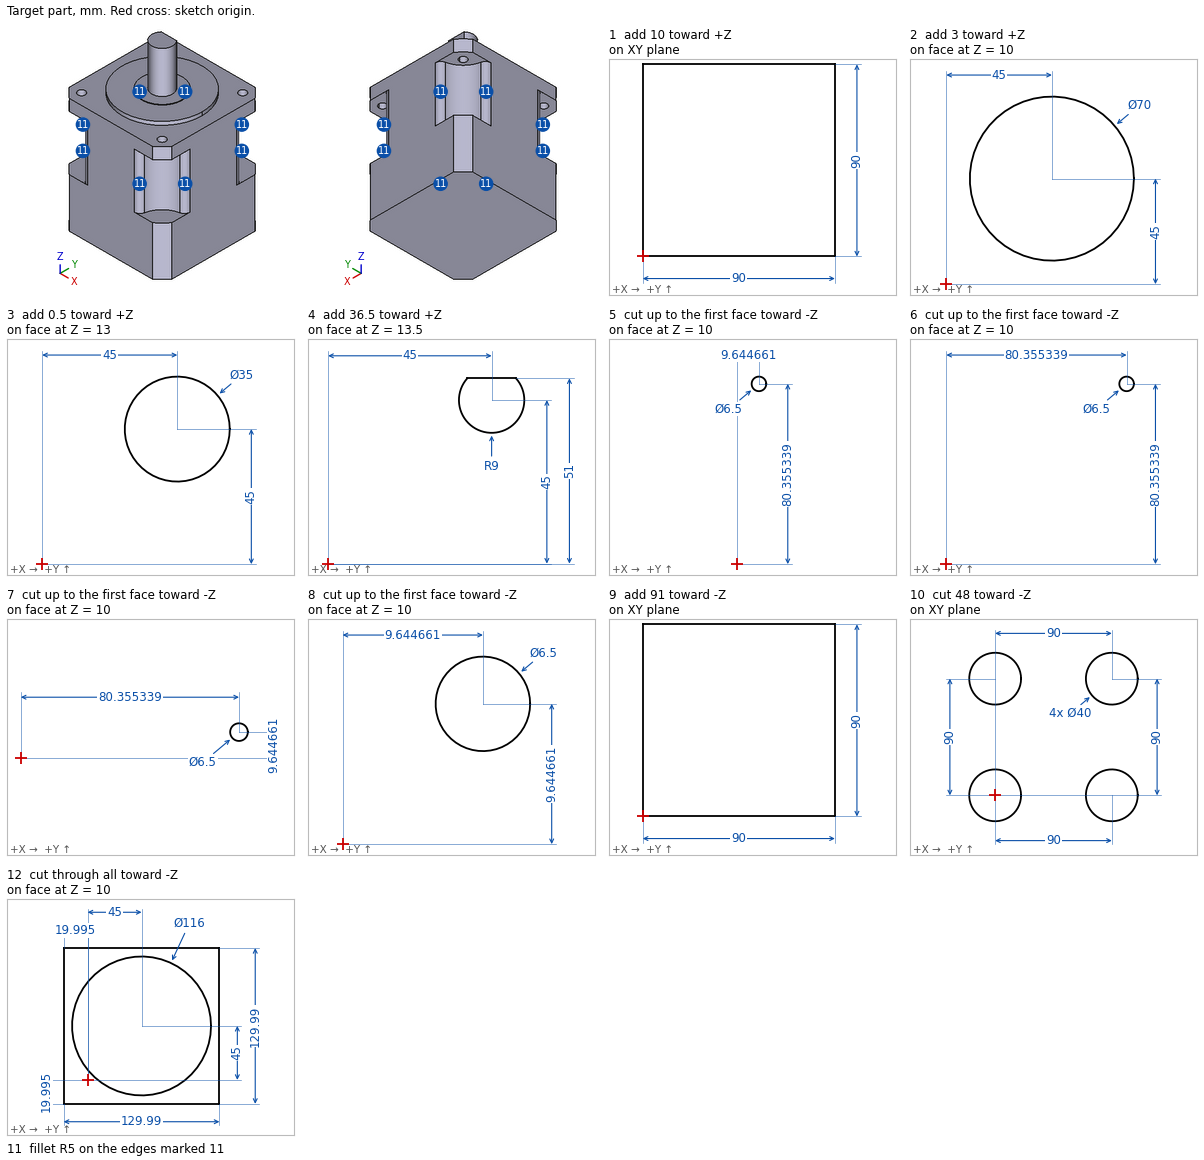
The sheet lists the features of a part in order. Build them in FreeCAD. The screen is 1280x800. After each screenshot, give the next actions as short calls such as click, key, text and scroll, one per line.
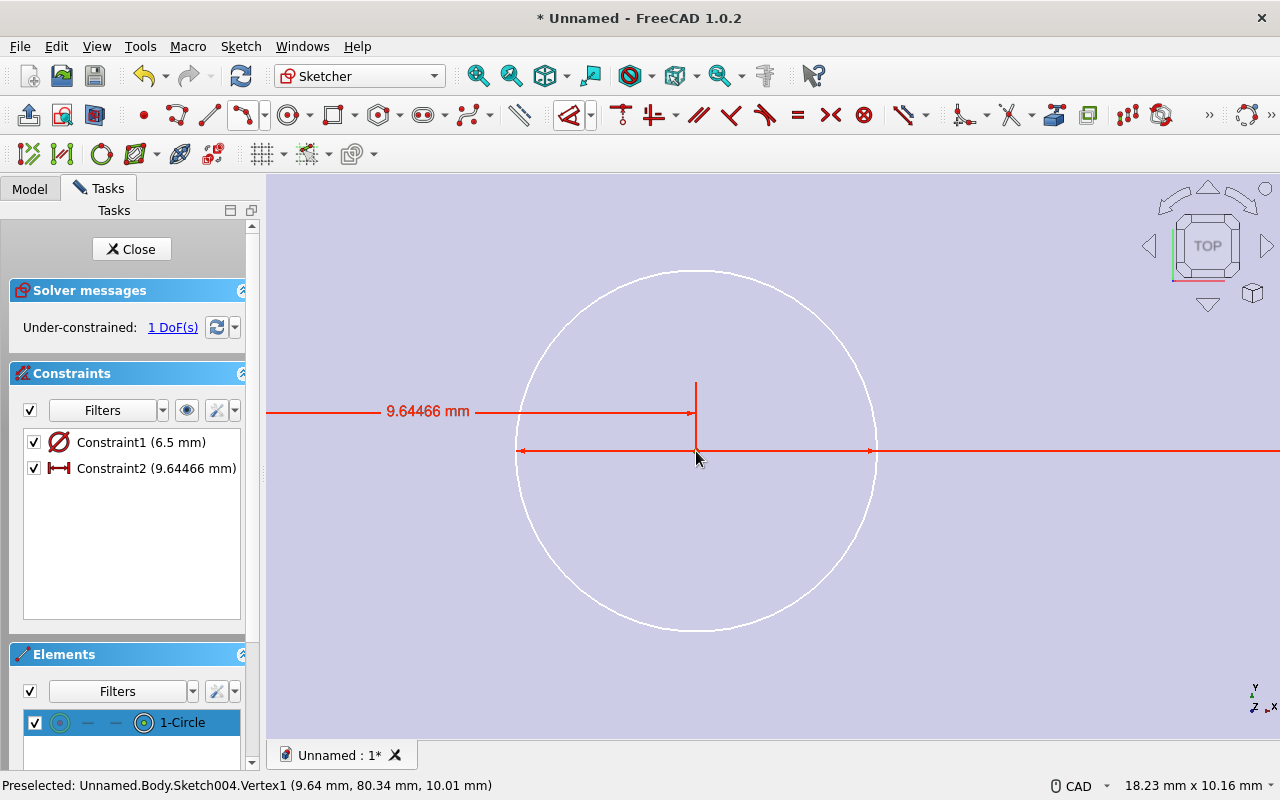
key(i)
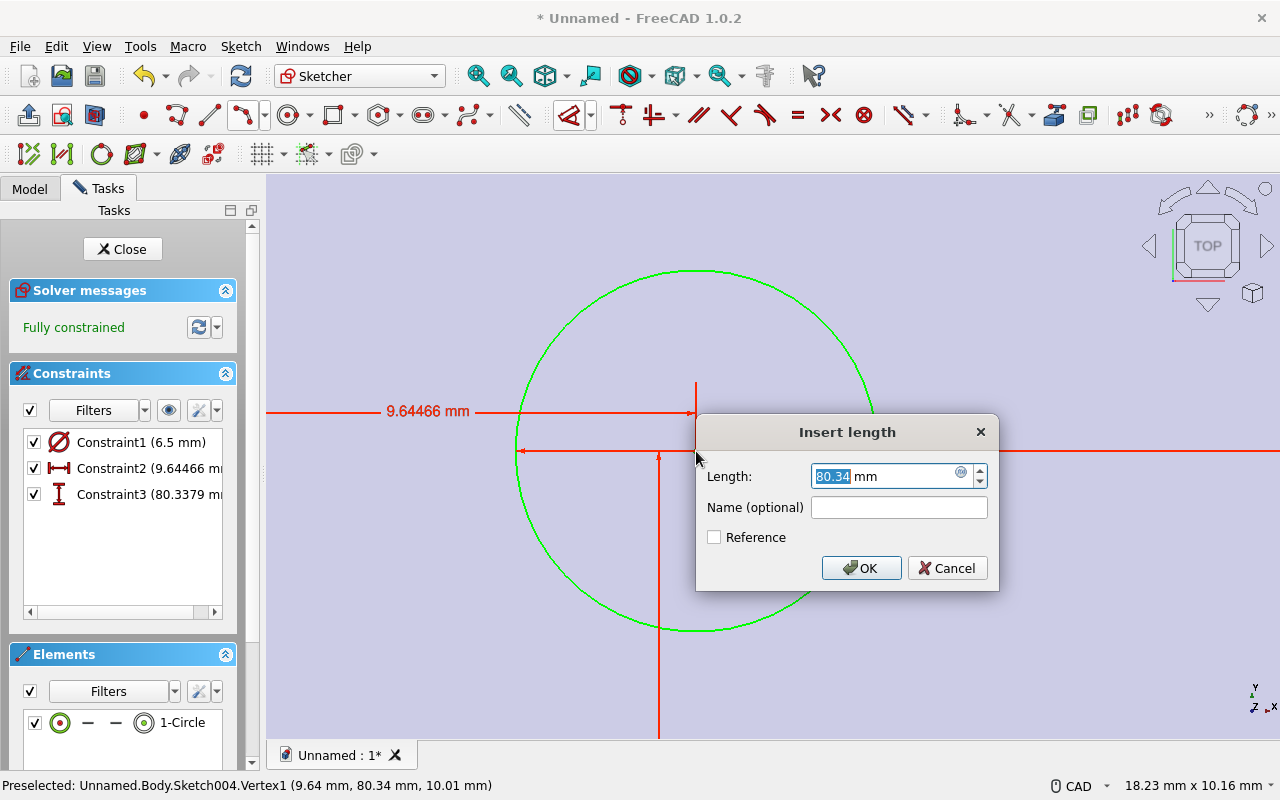
text(80.355339)
key(Return)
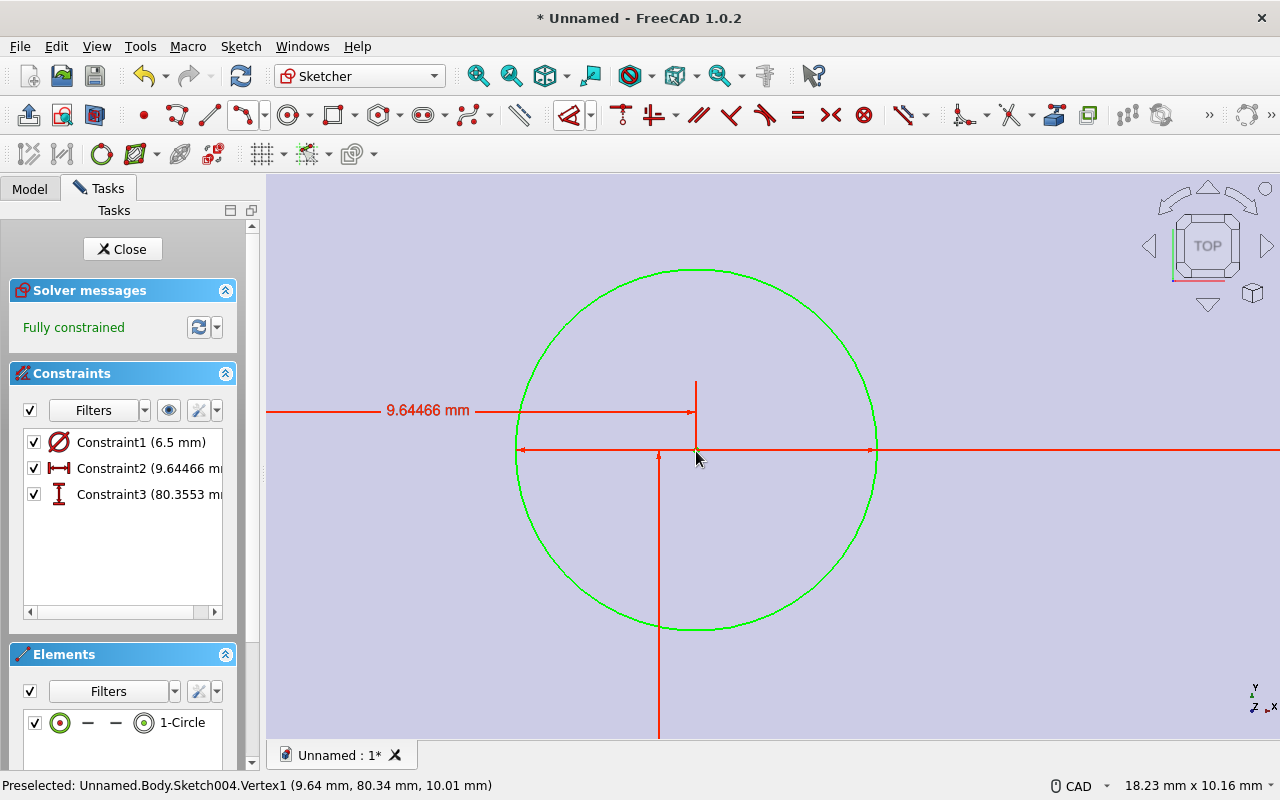
click(123, 249)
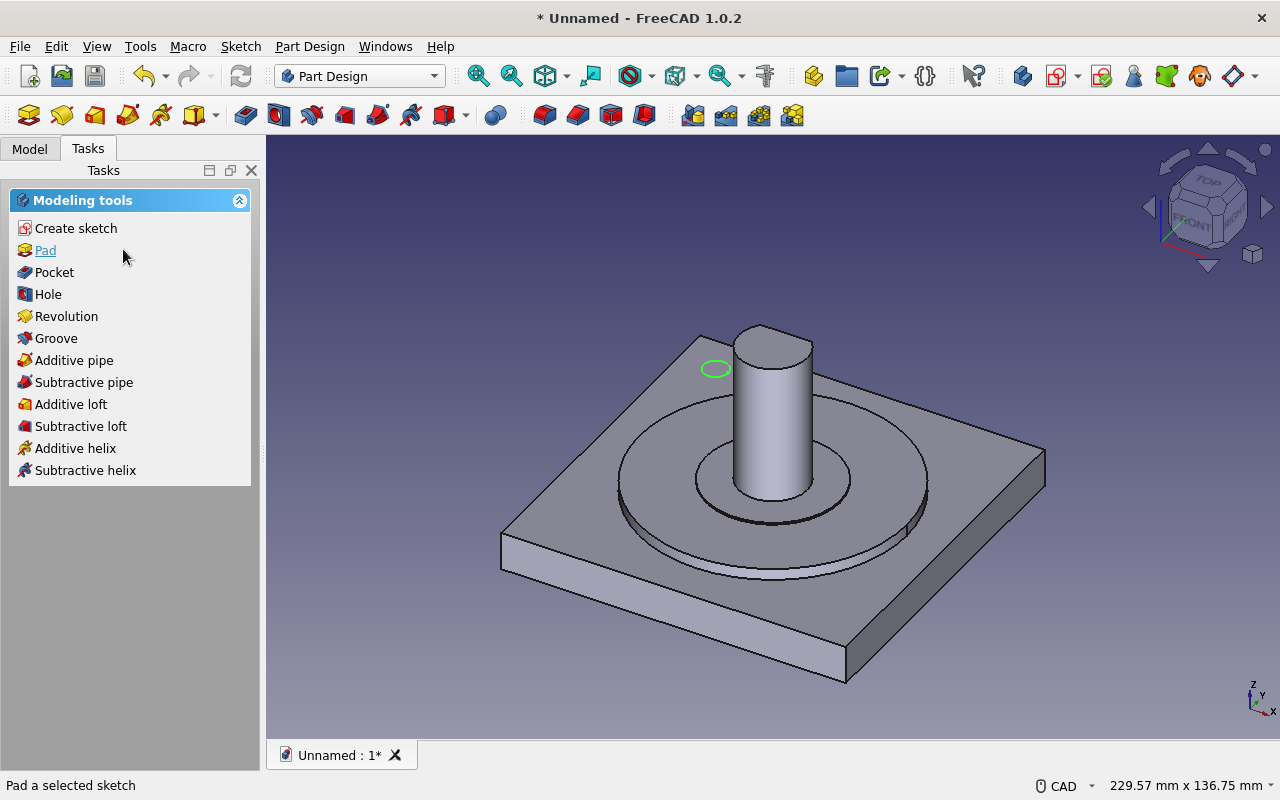
click(246, 116)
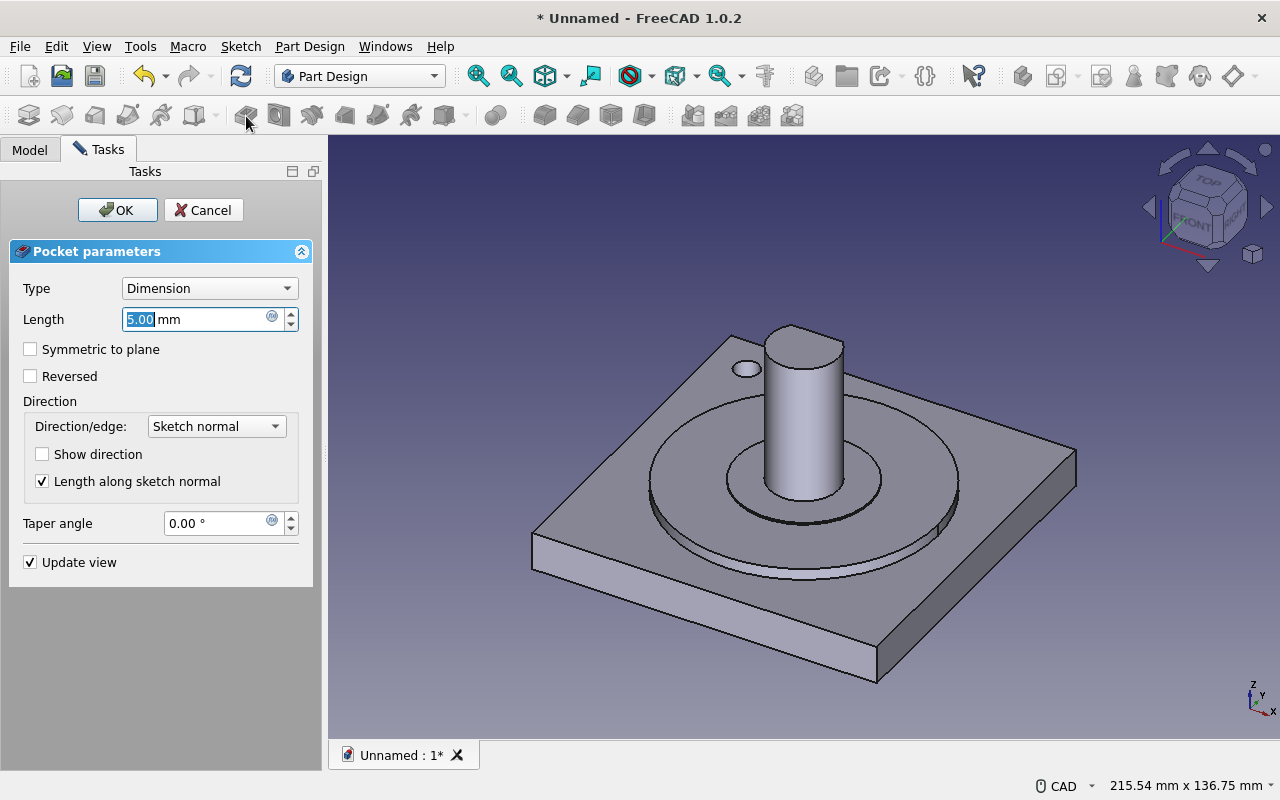
click(210, 288)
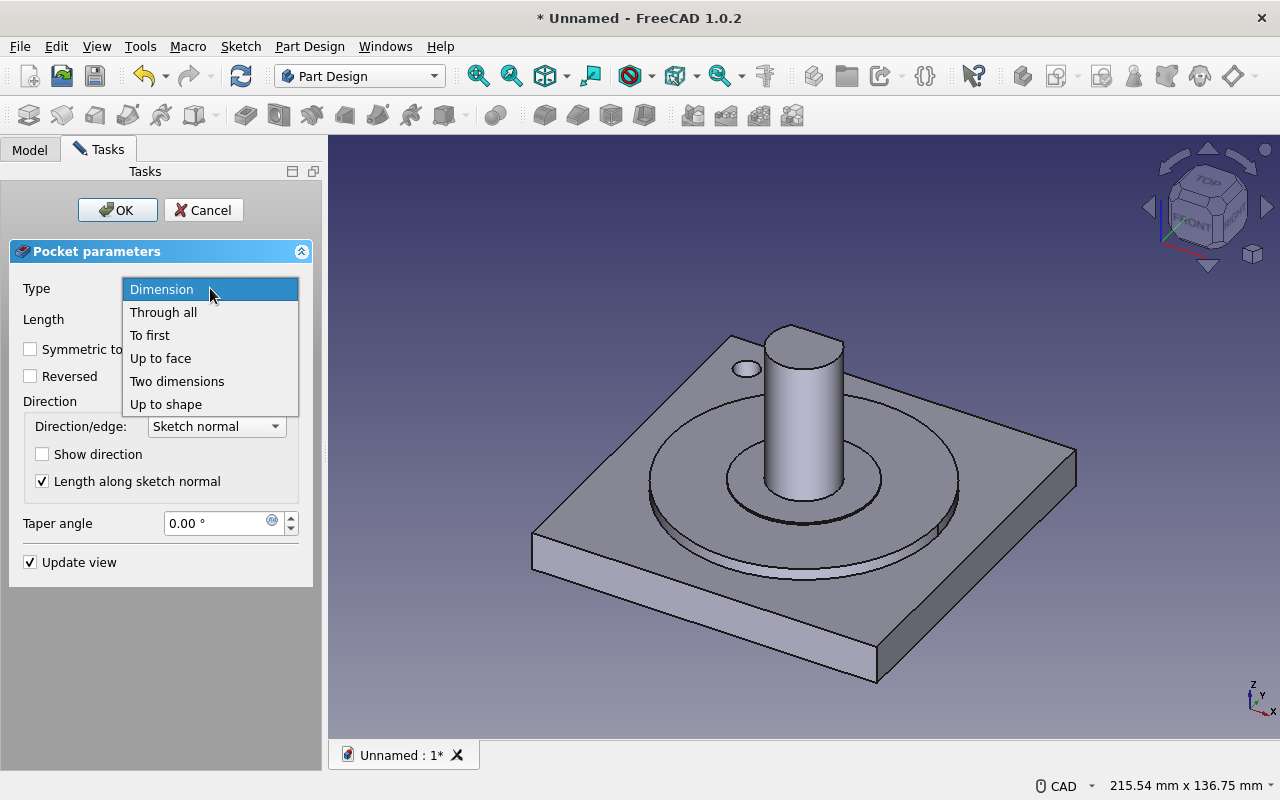
click(208, 336)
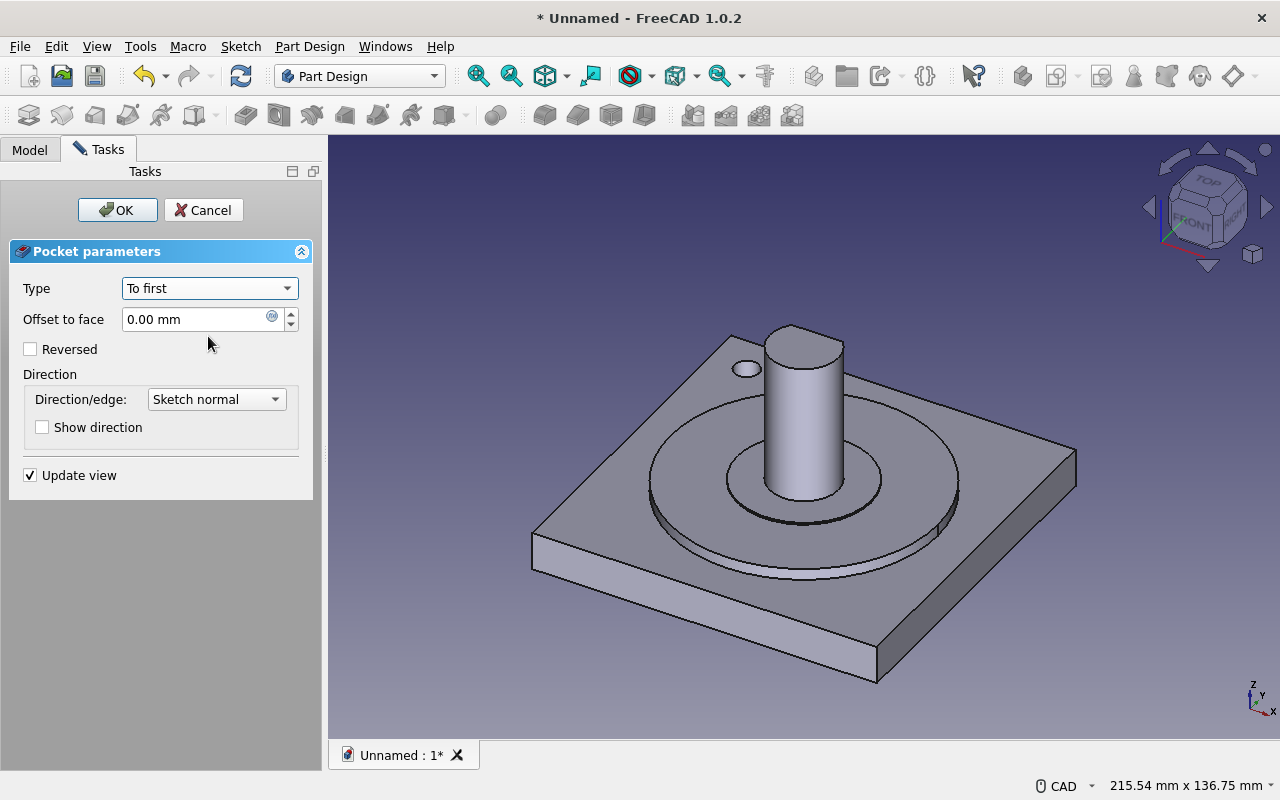
click(118, 210)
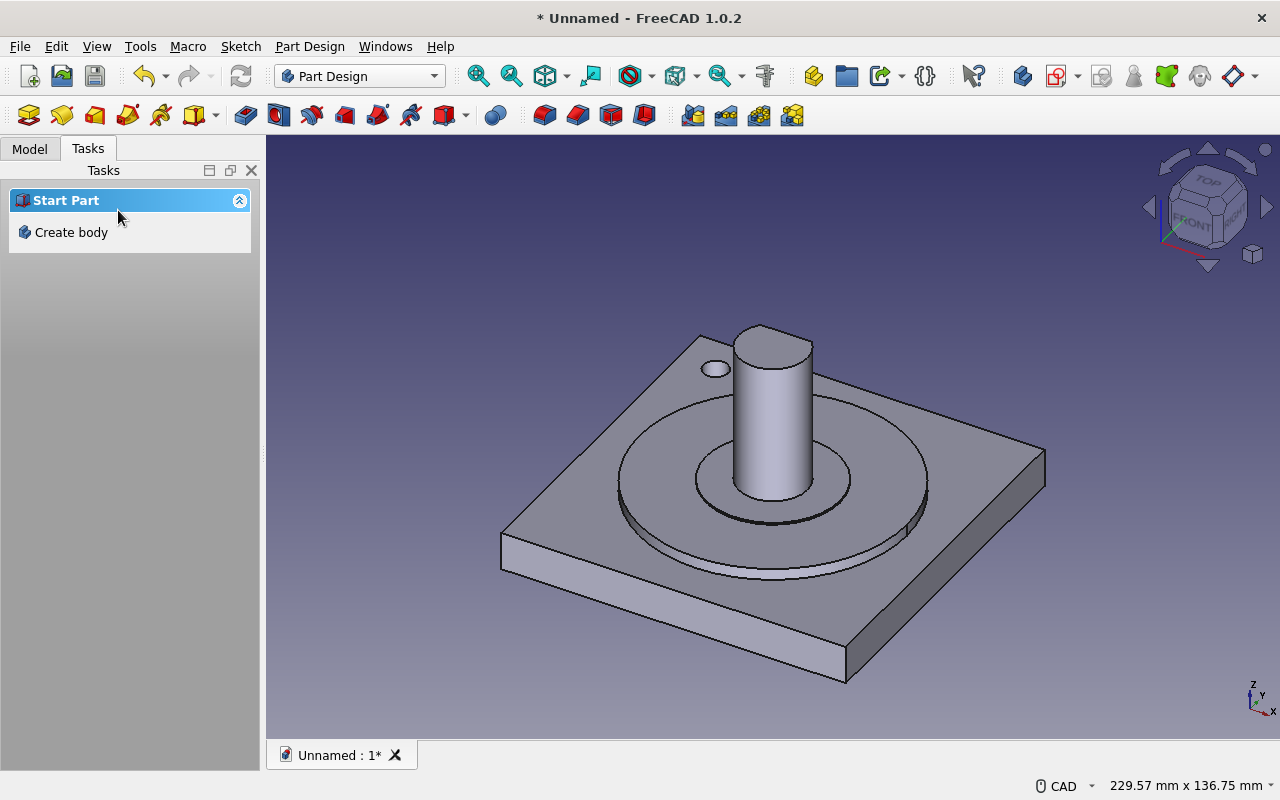
click(1006, 455)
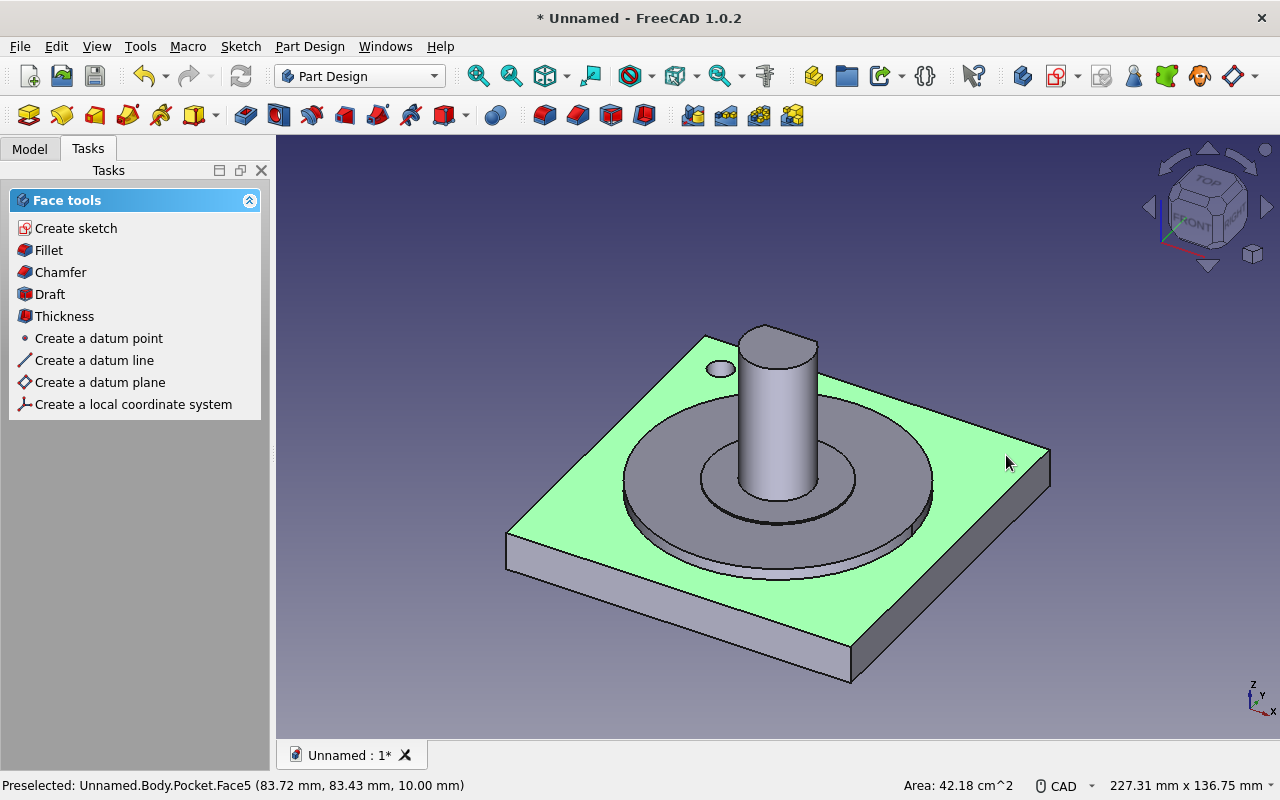
click(1056, 76)